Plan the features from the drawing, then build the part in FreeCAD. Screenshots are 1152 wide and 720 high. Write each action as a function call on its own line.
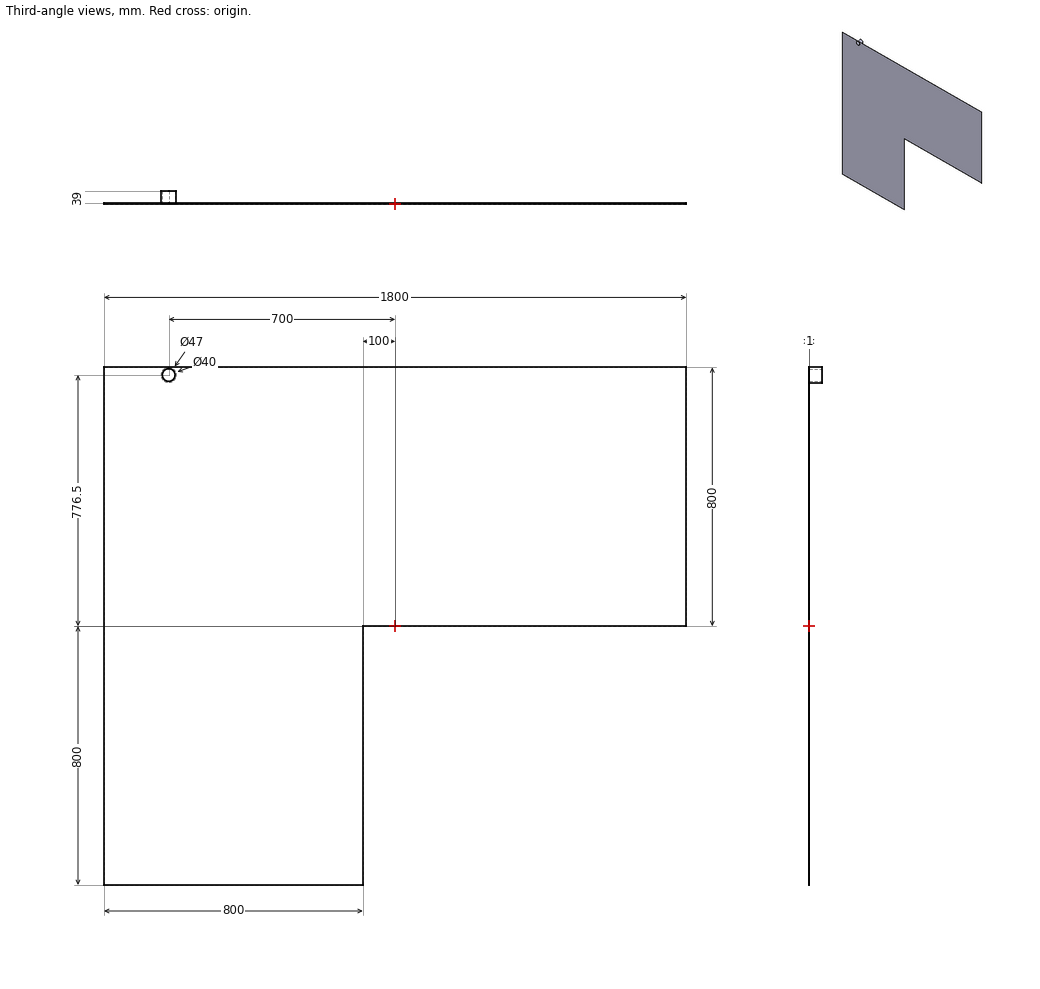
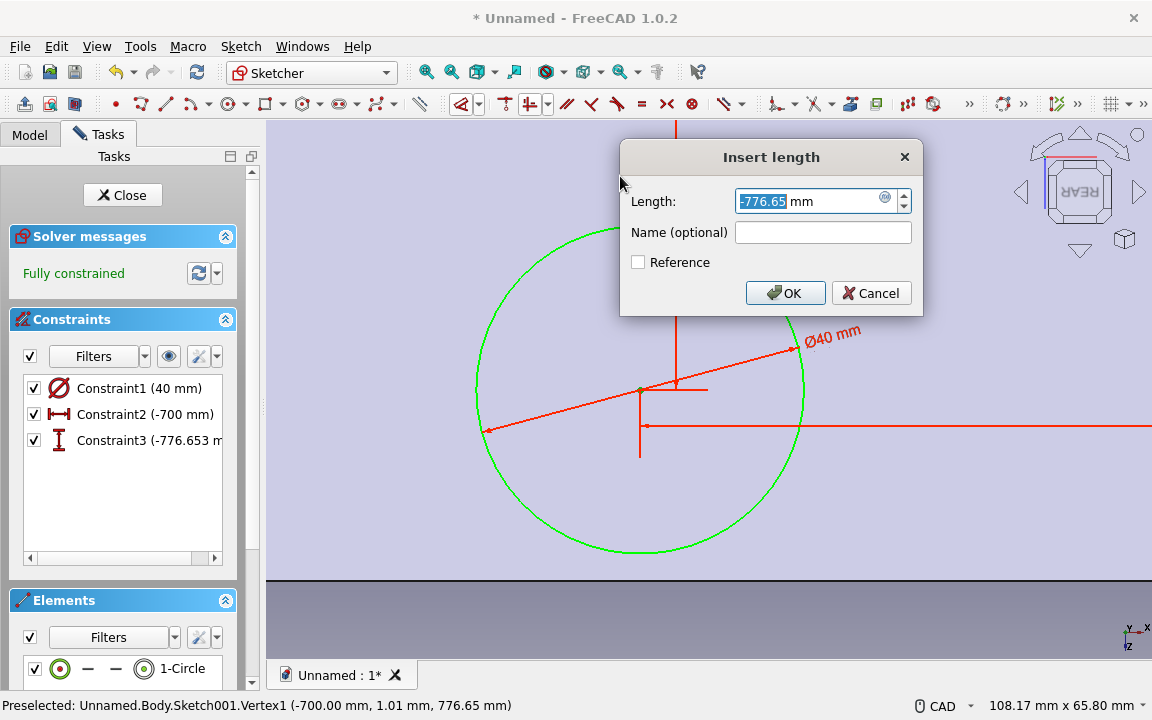
text(-776.5)
key(Return)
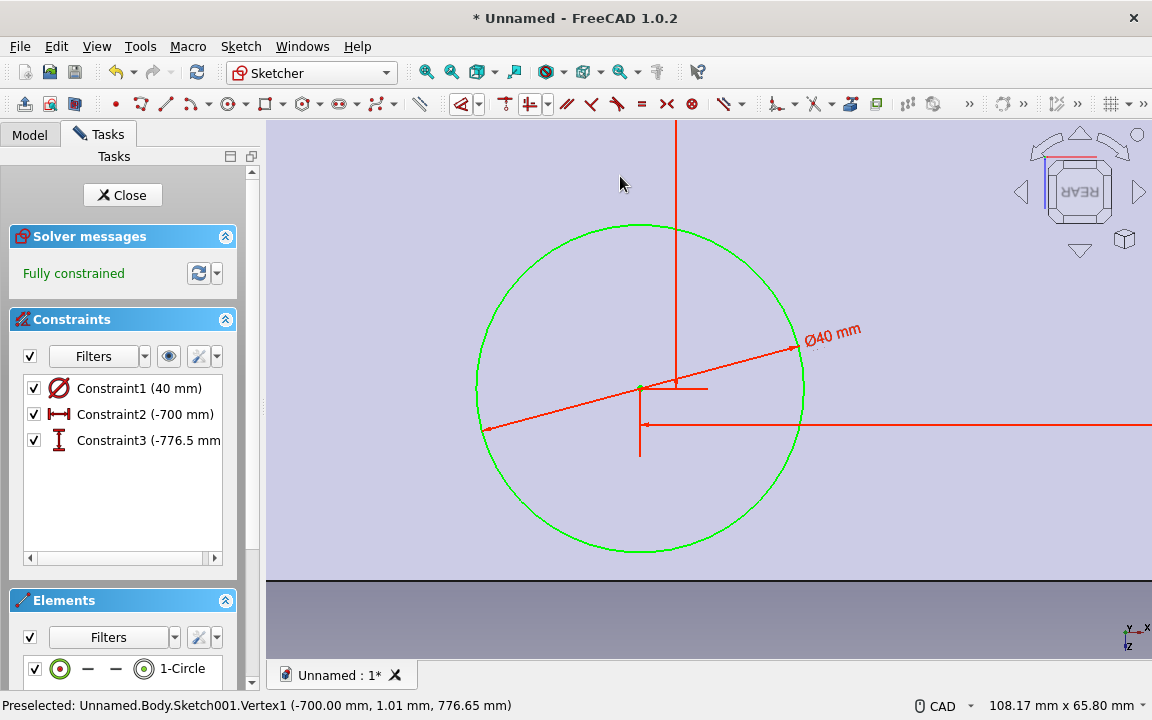
click(123, 195)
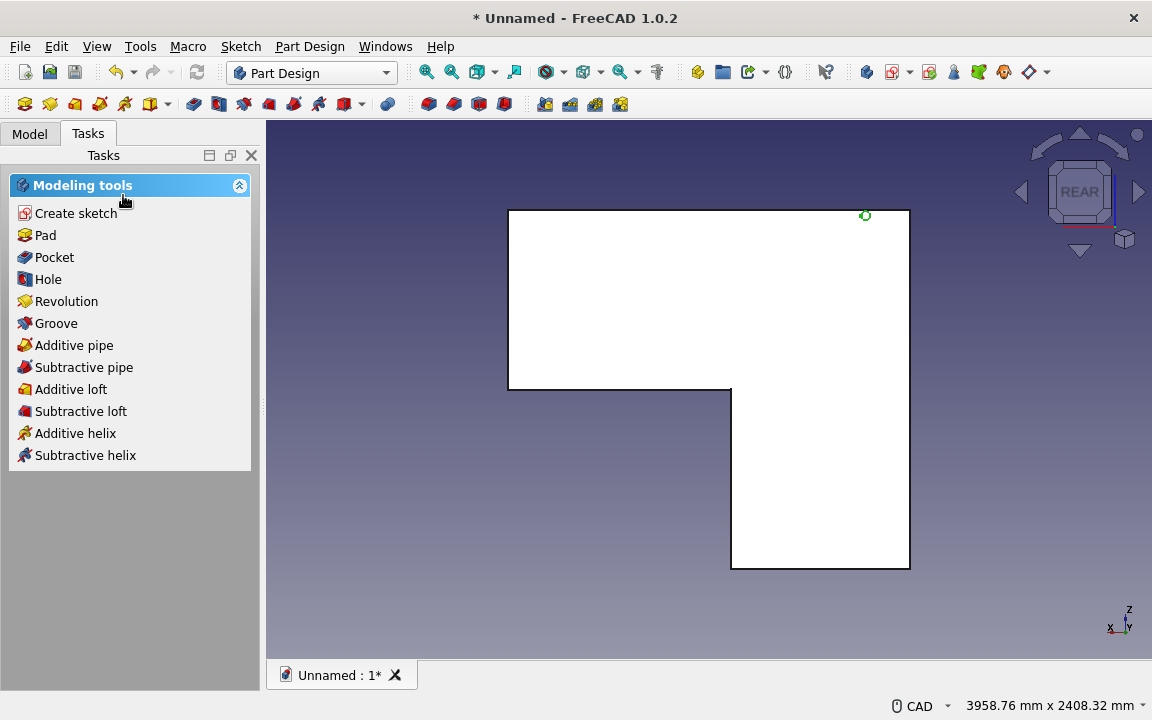
click(194, 104)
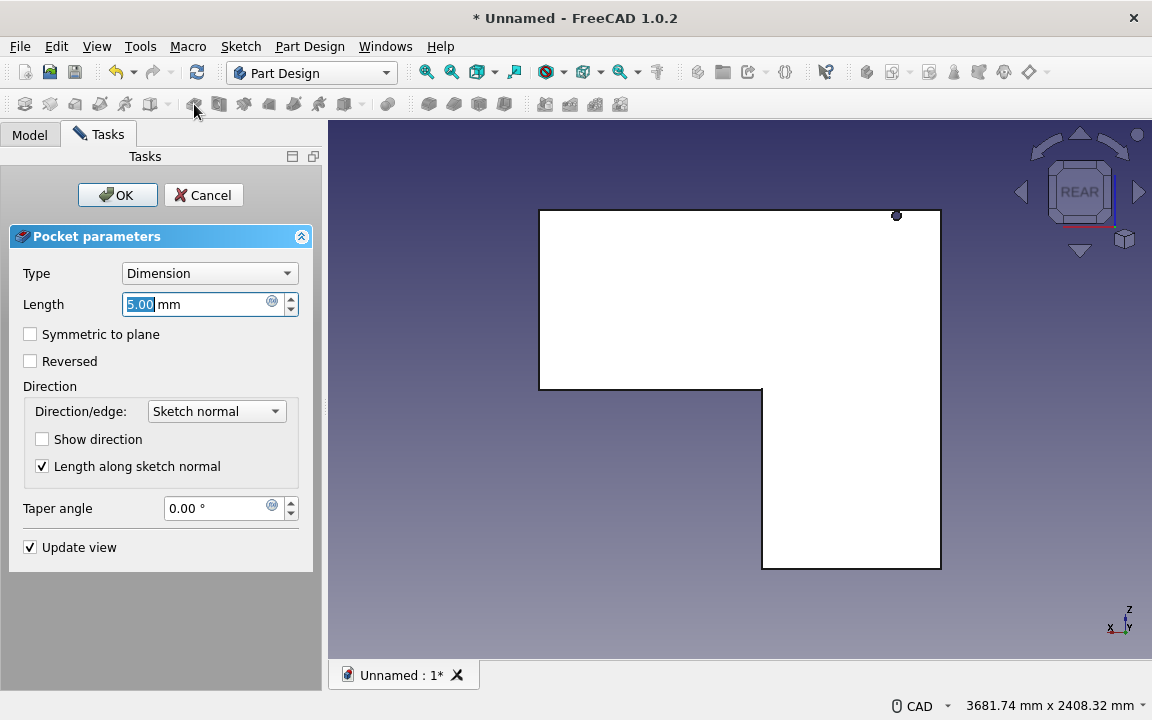
click(210, 274)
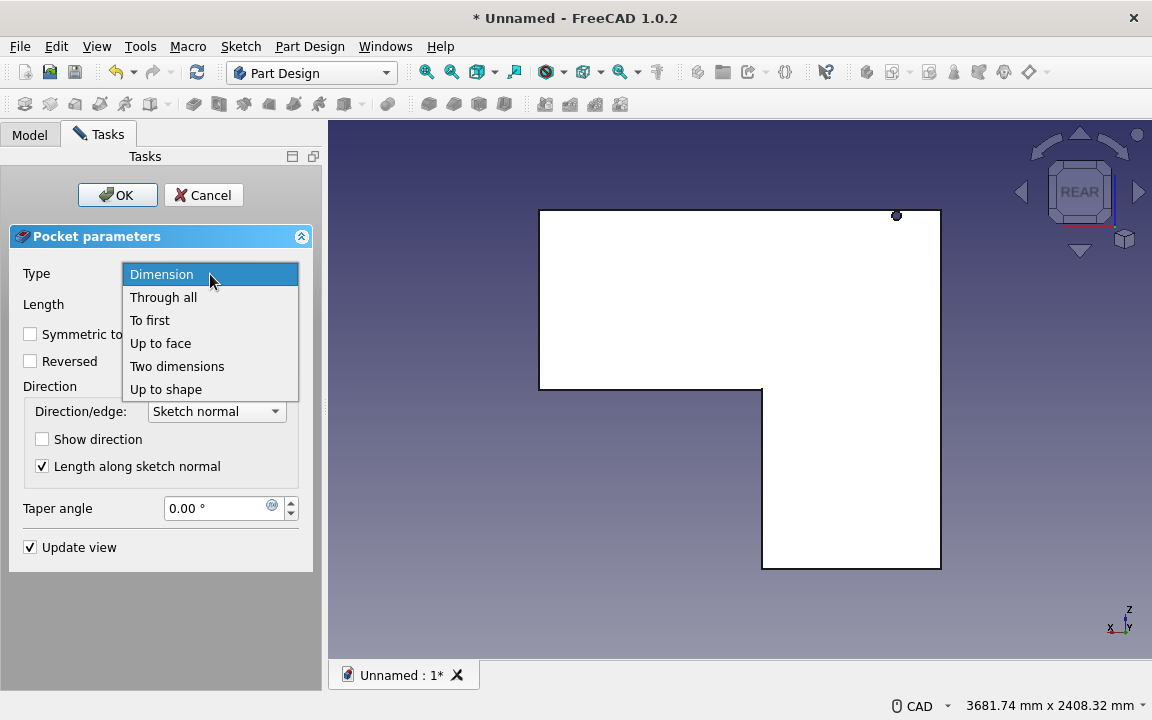
click(208, 298)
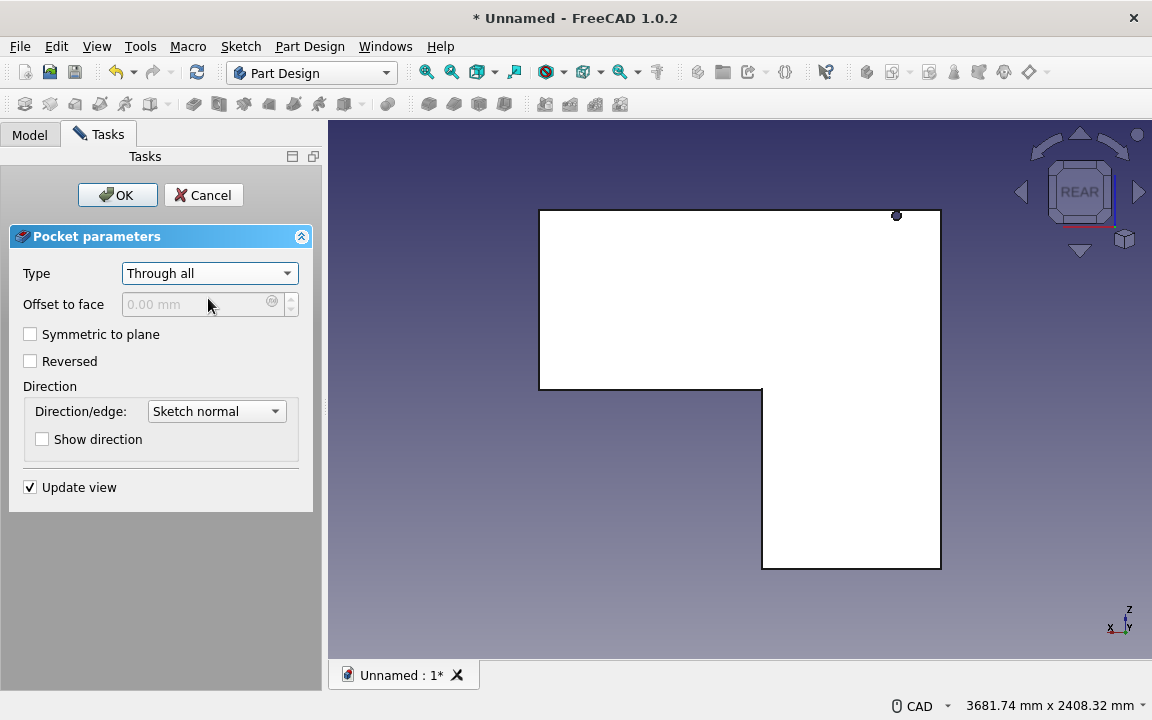
click(118, 195)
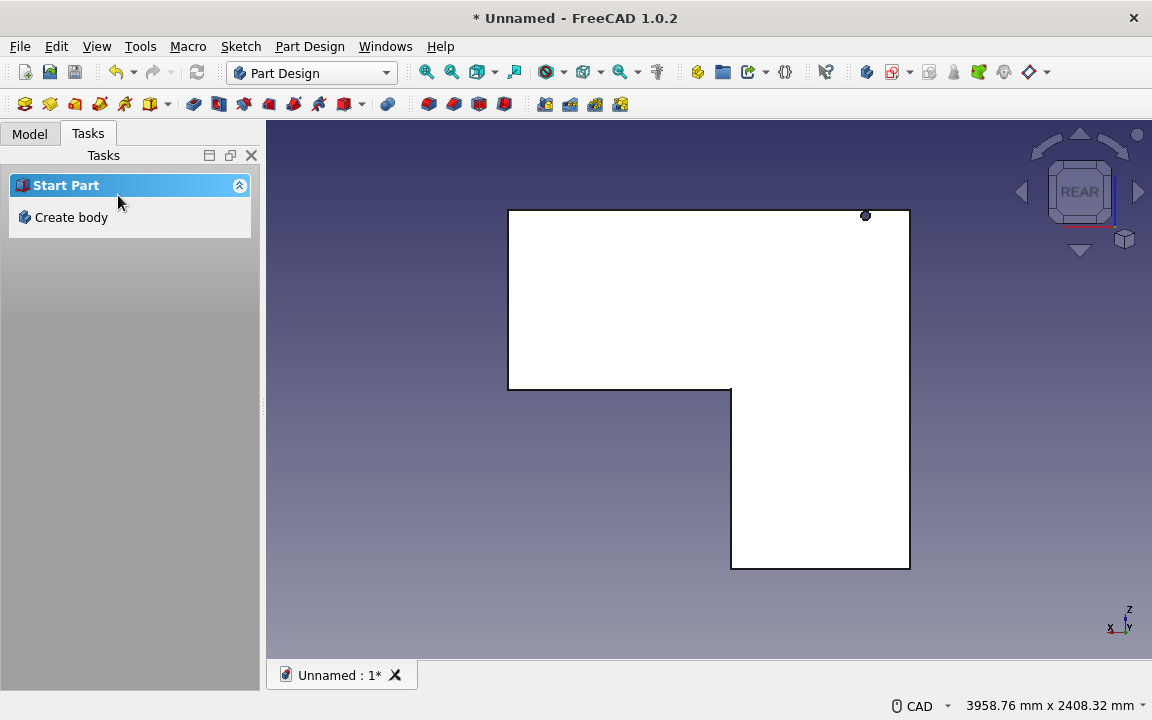
click(30, 134)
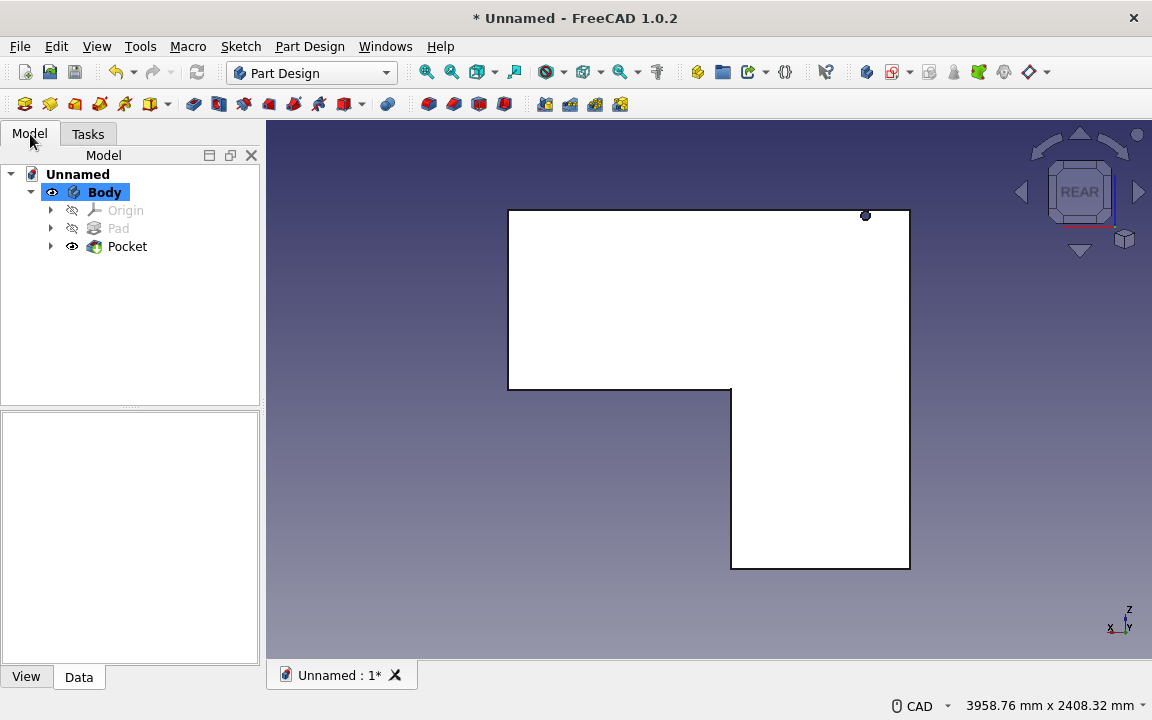
click(51, 210)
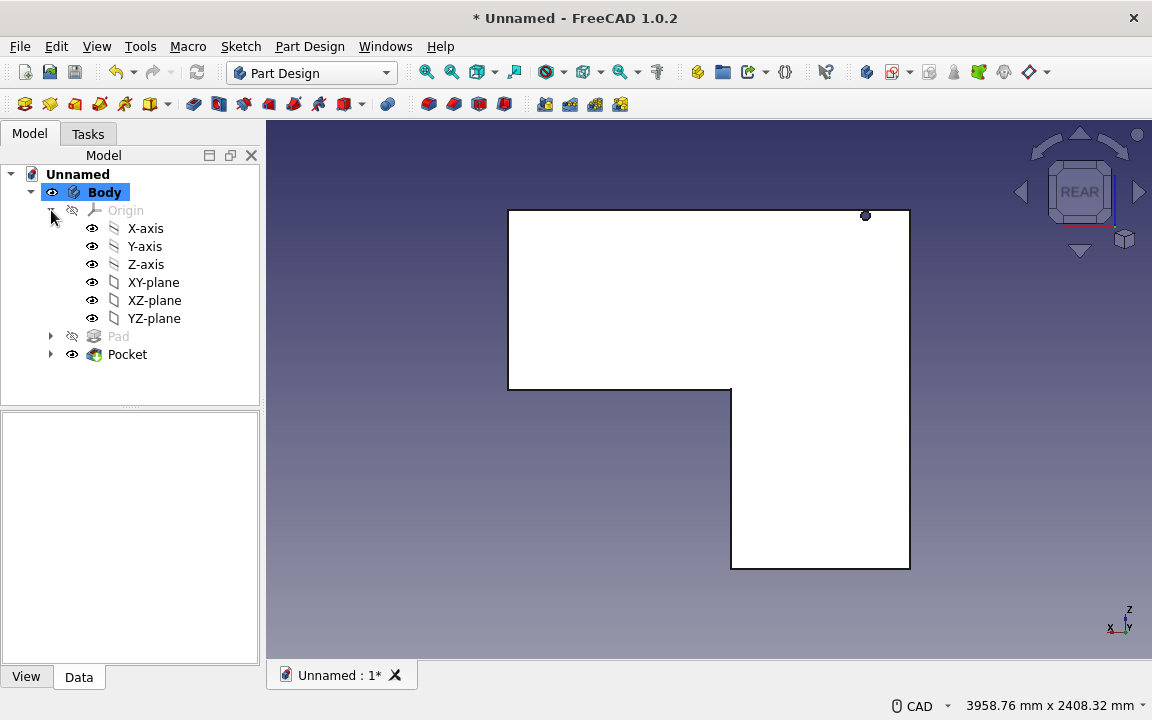
click(137, 300)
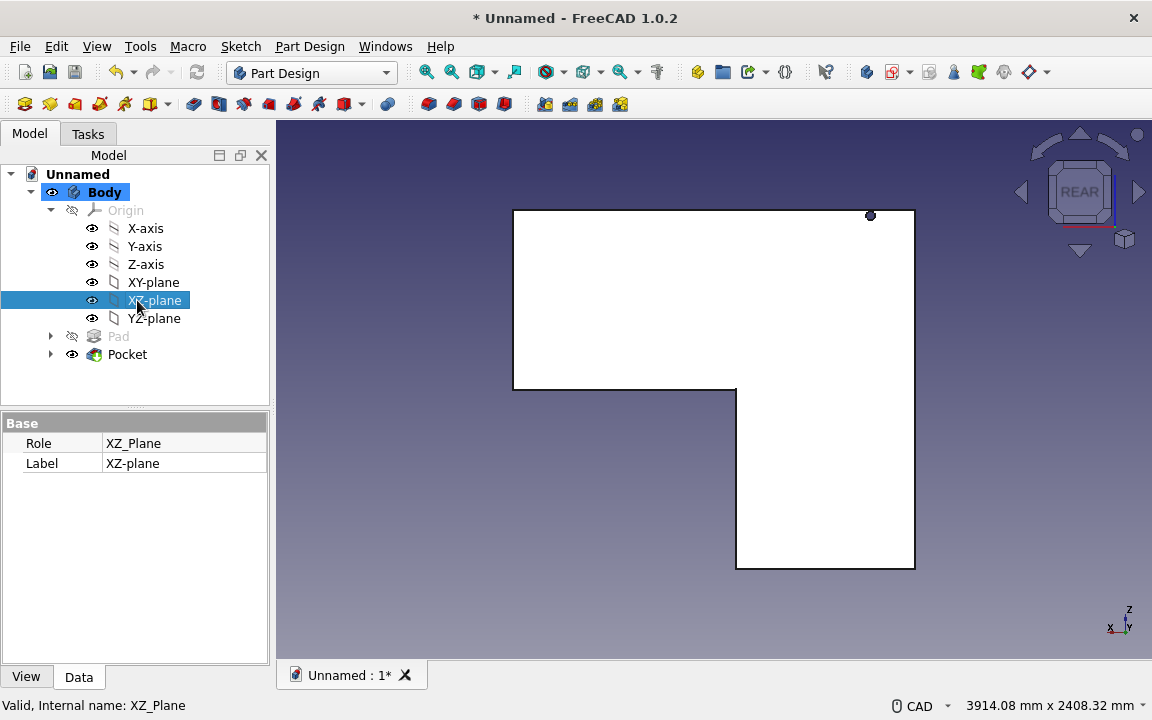
click(1028, 72)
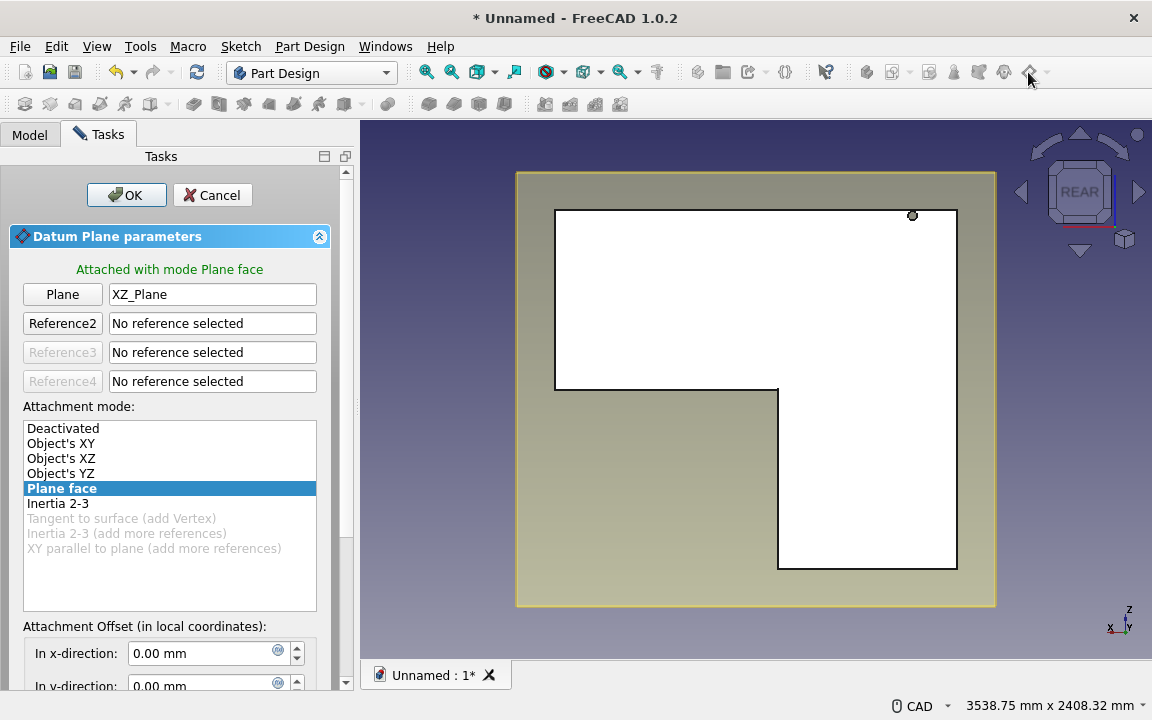
scroll(346, 428, down, 2)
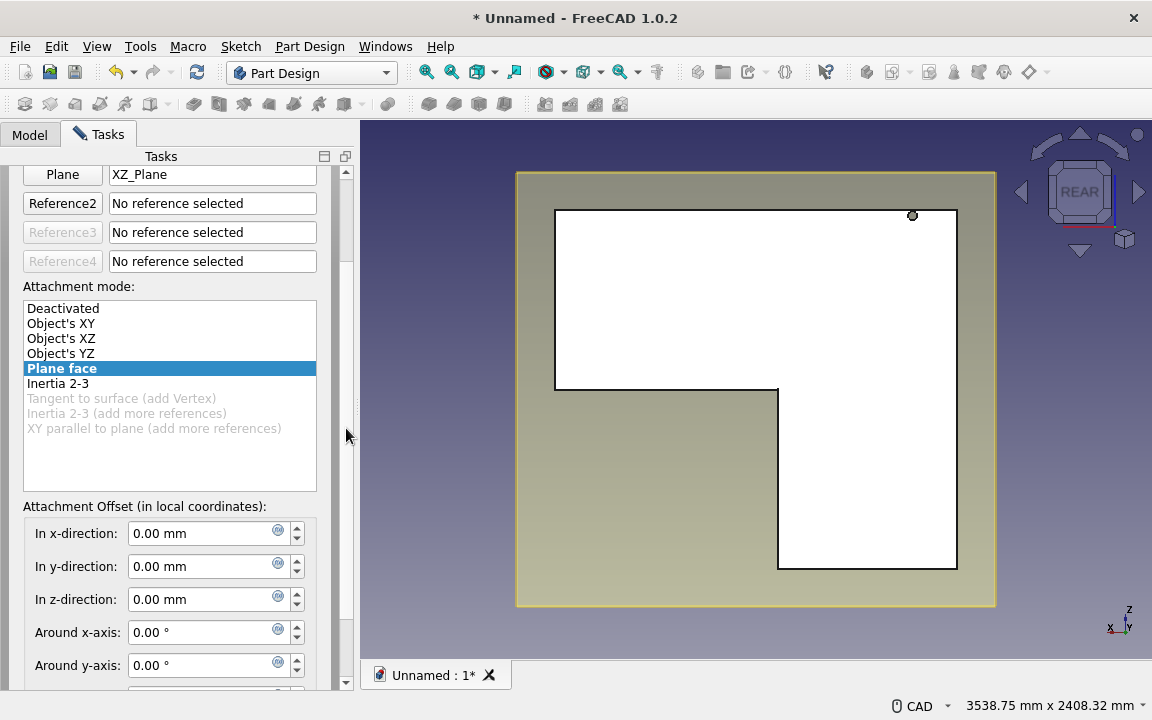
triple_click(210, 600)